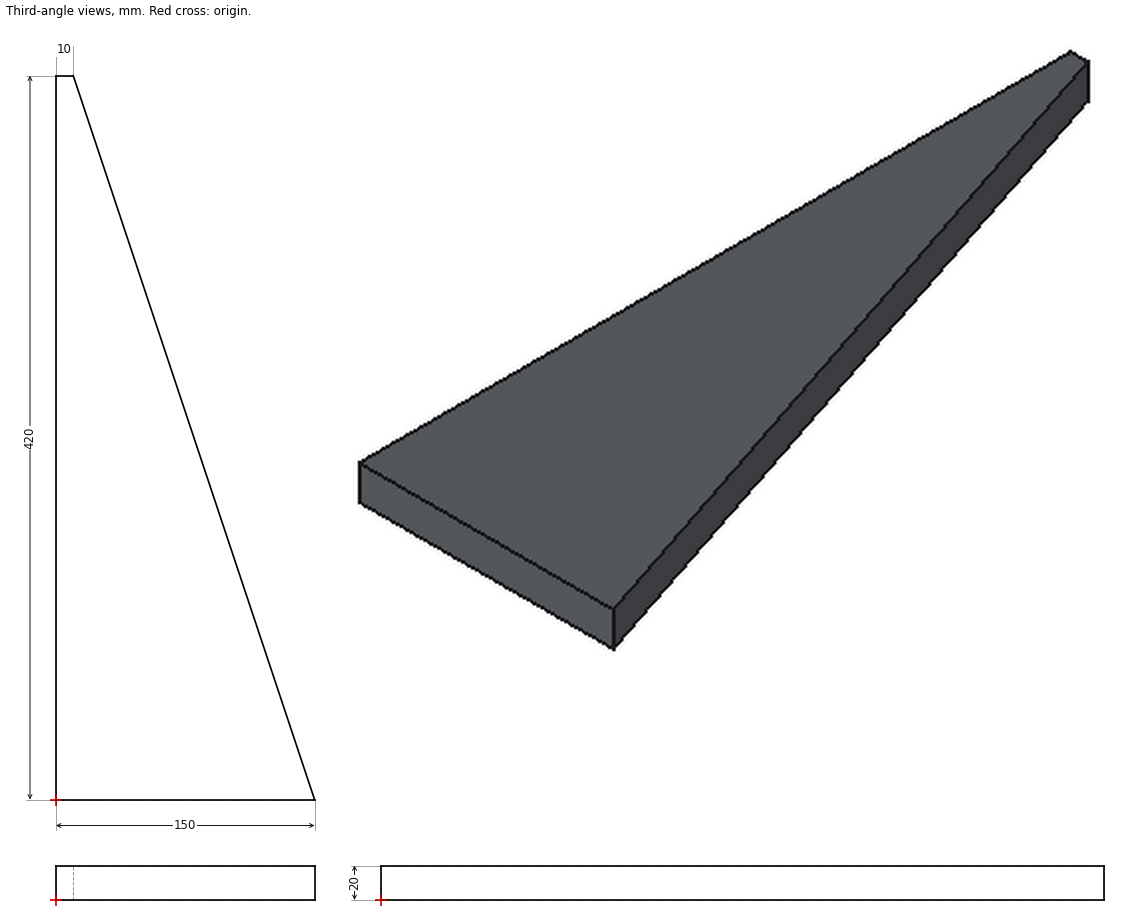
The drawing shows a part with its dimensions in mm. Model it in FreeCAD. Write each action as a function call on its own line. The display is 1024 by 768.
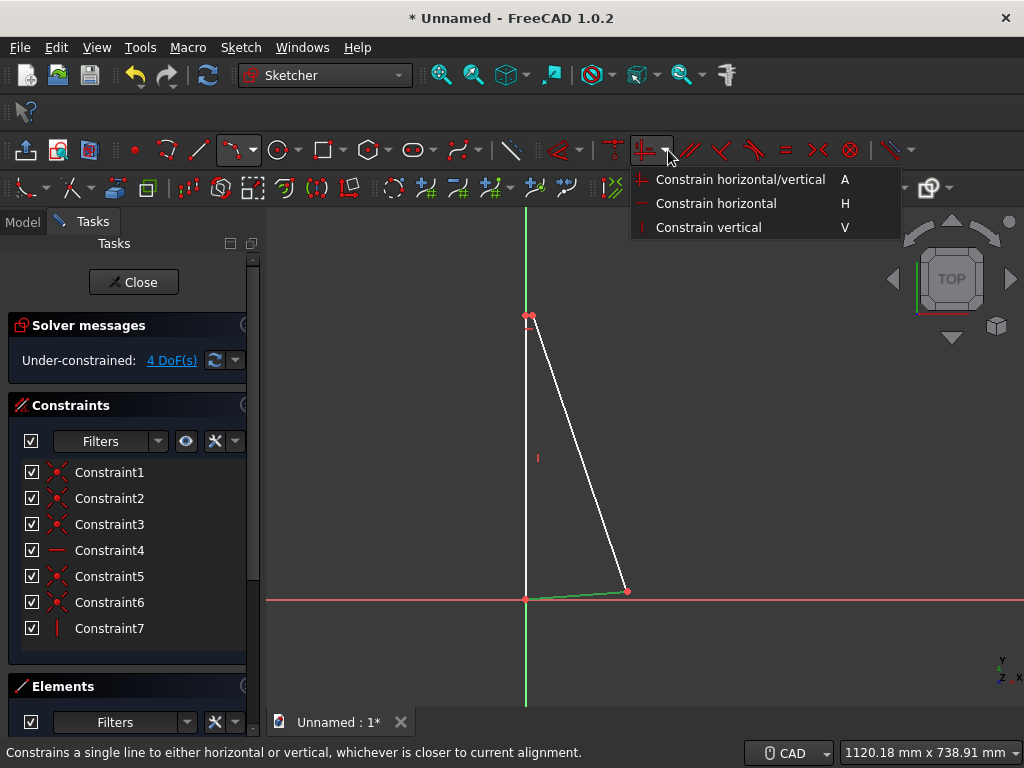
click(766, 203)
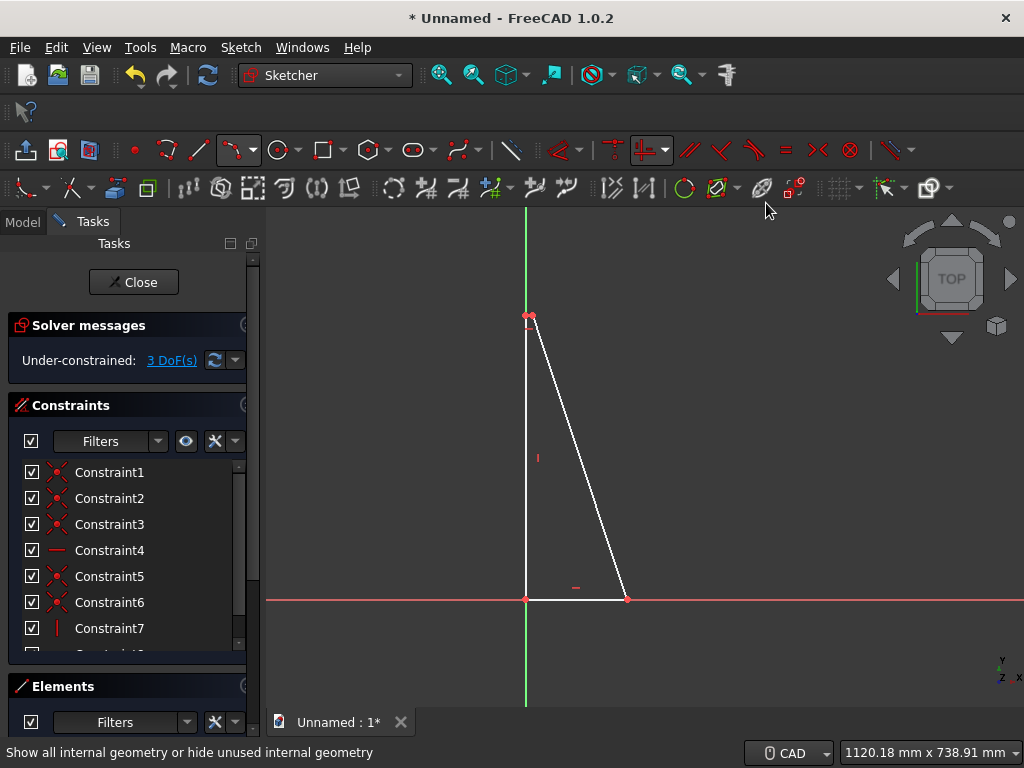
click(558, 150)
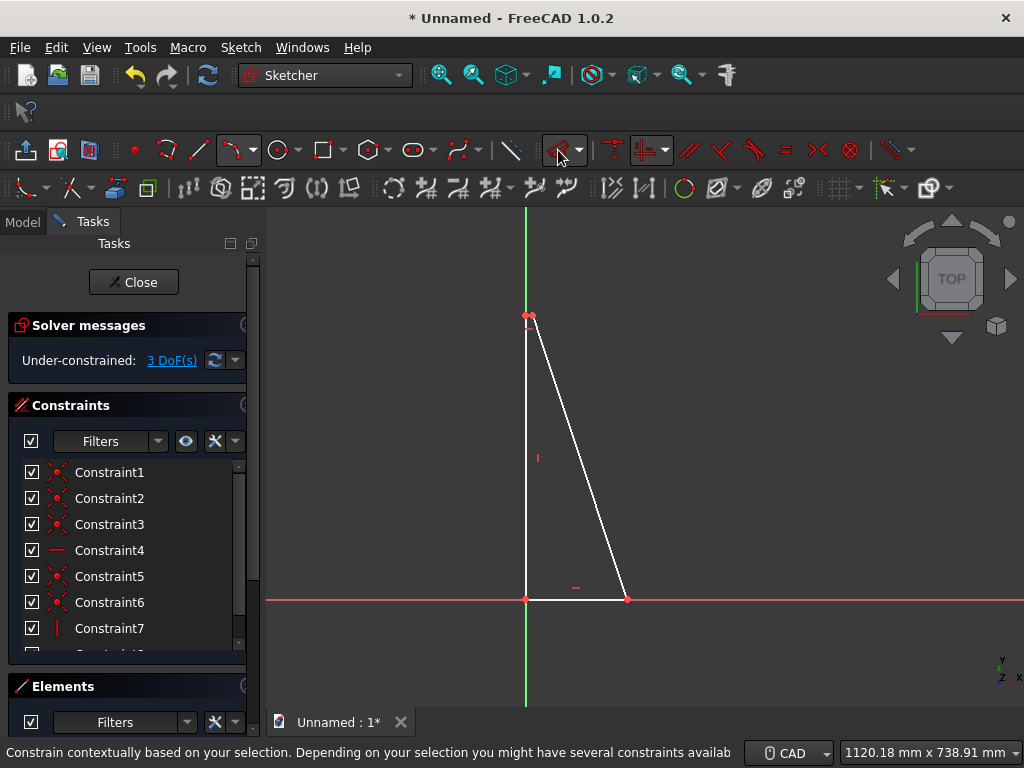
scroll(529, 316, up, 9)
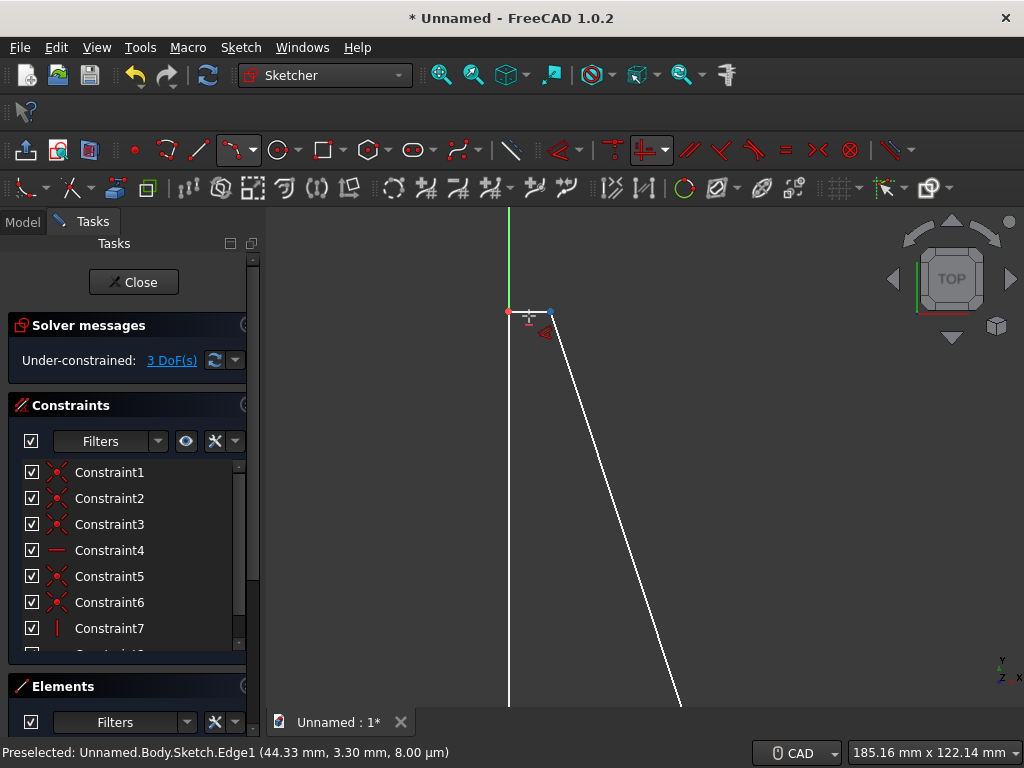
click(530, 312)
click(530, 278)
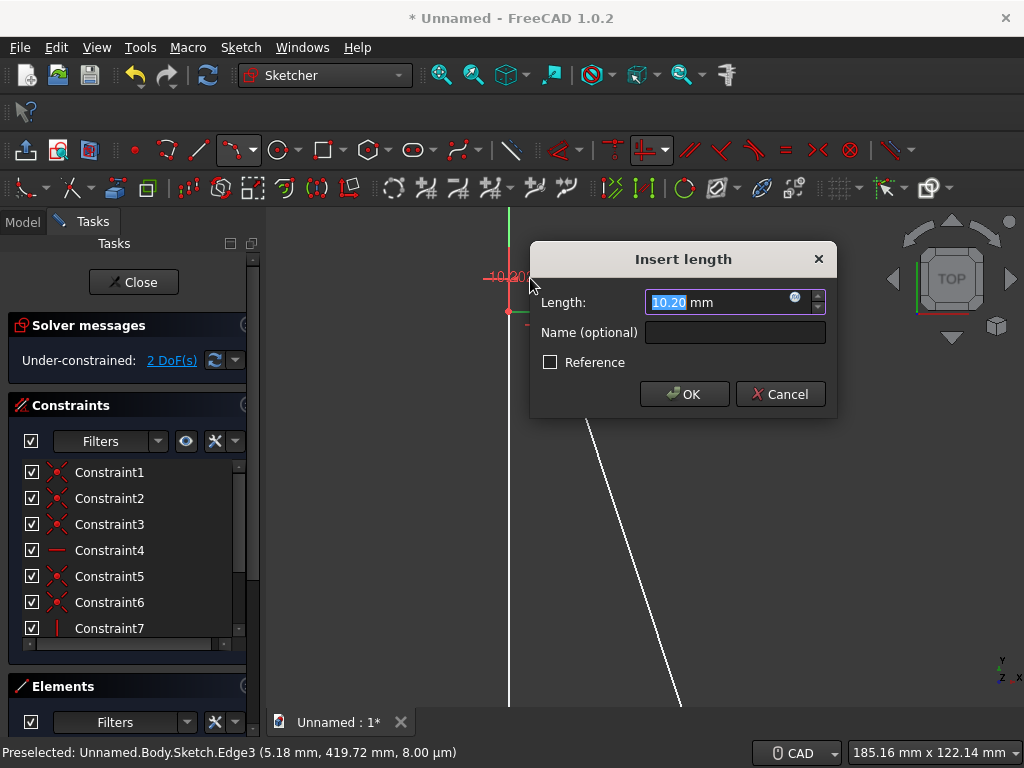
text(10)
key(Return)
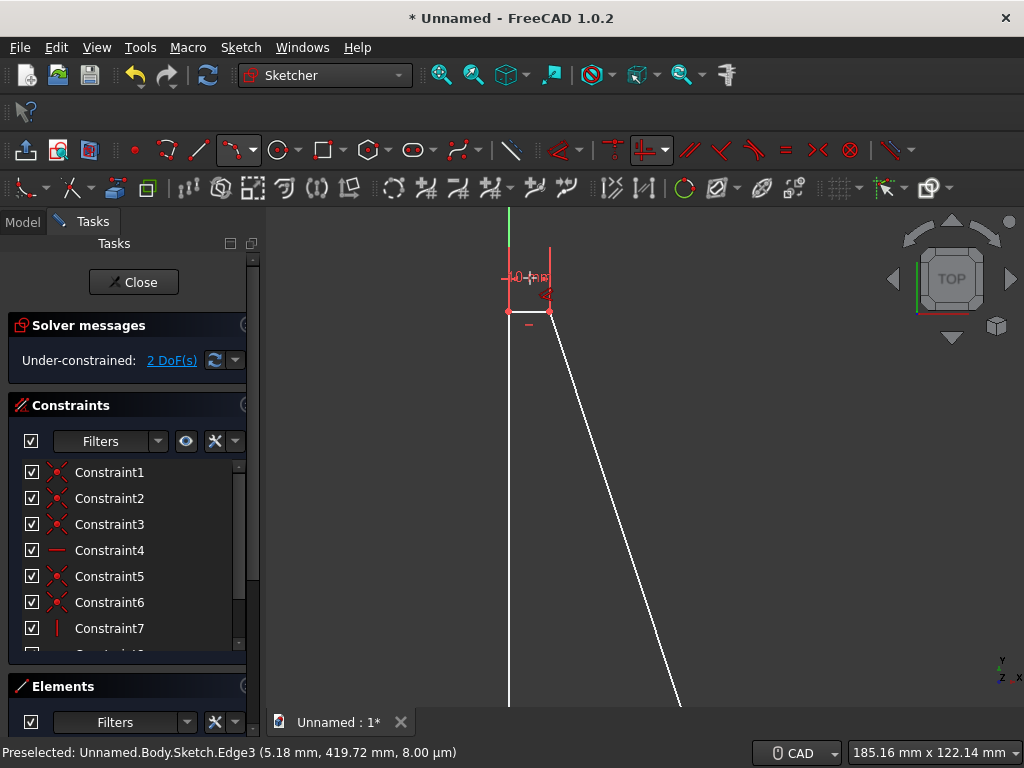
scroll(529, 316, down, 9)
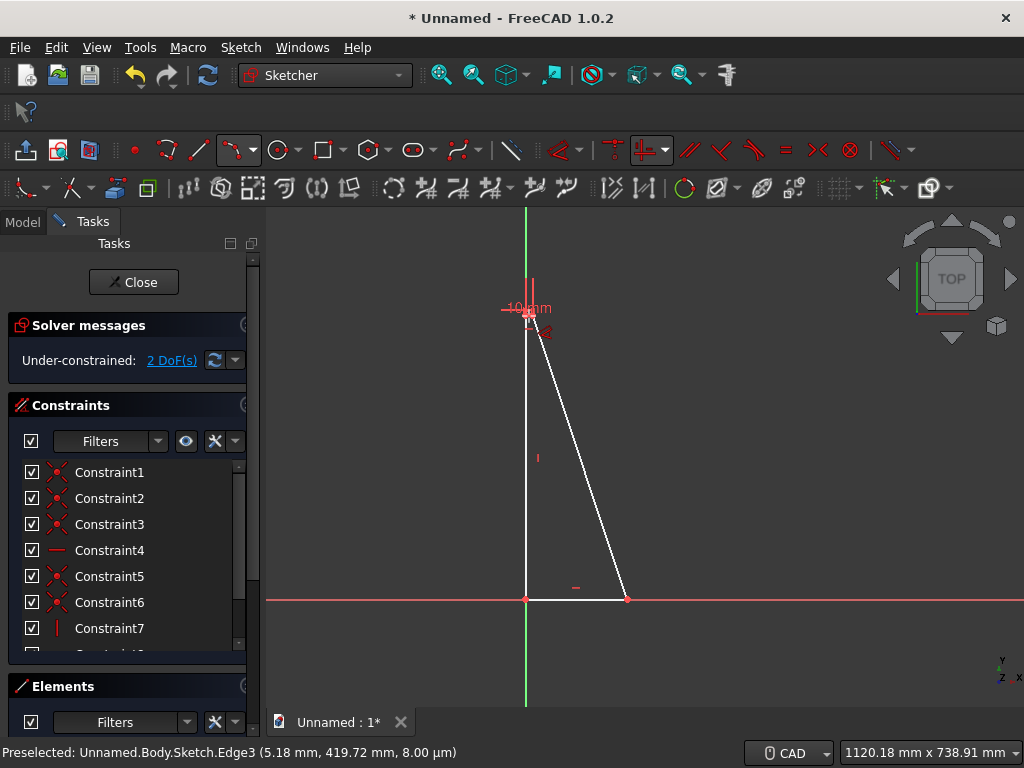
click(556, 600)
click(576, 634)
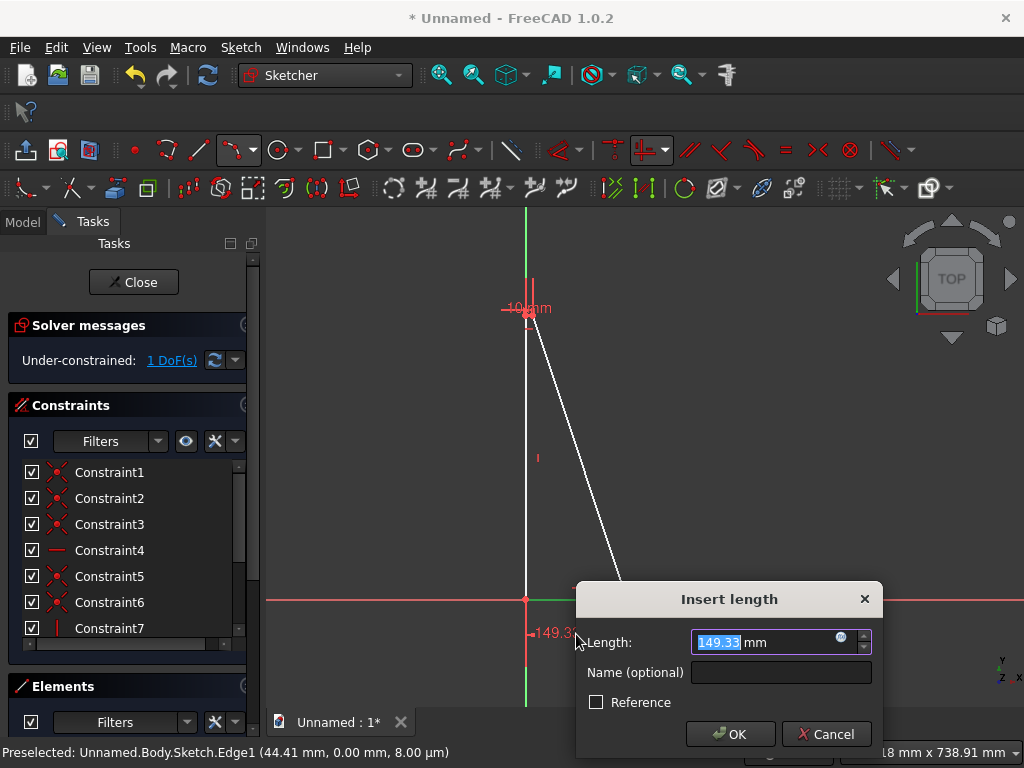
text(150)
key(Return)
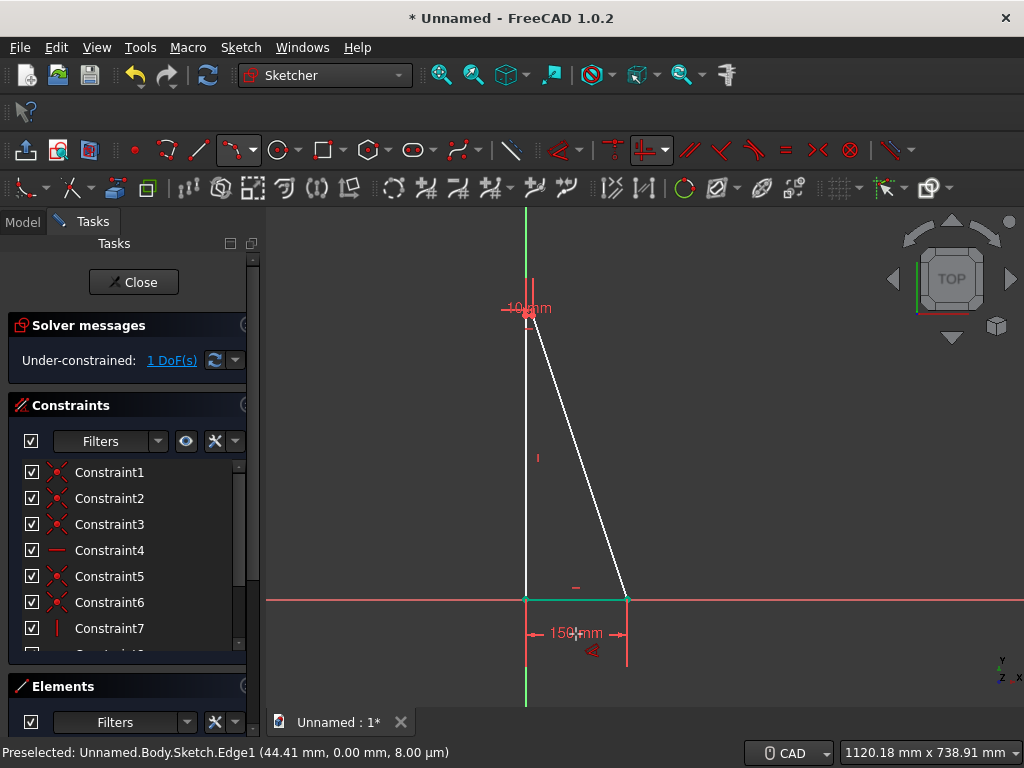
click(526, 401)
click(492, 458)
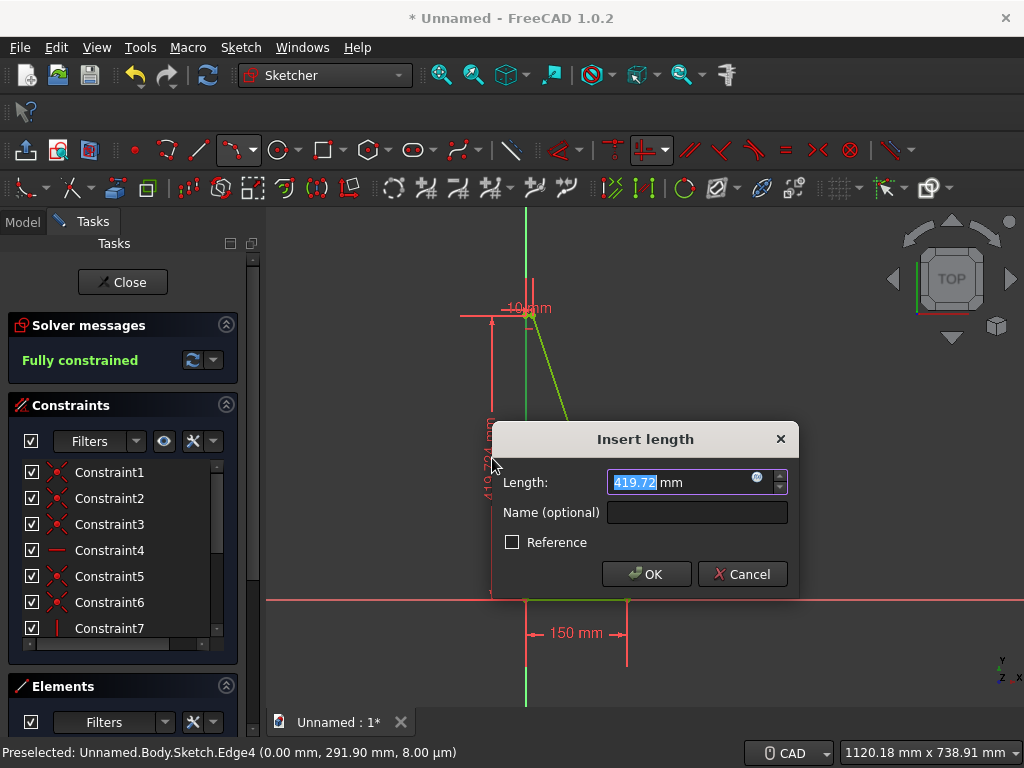
text(420)
key(Return)
key(Escape)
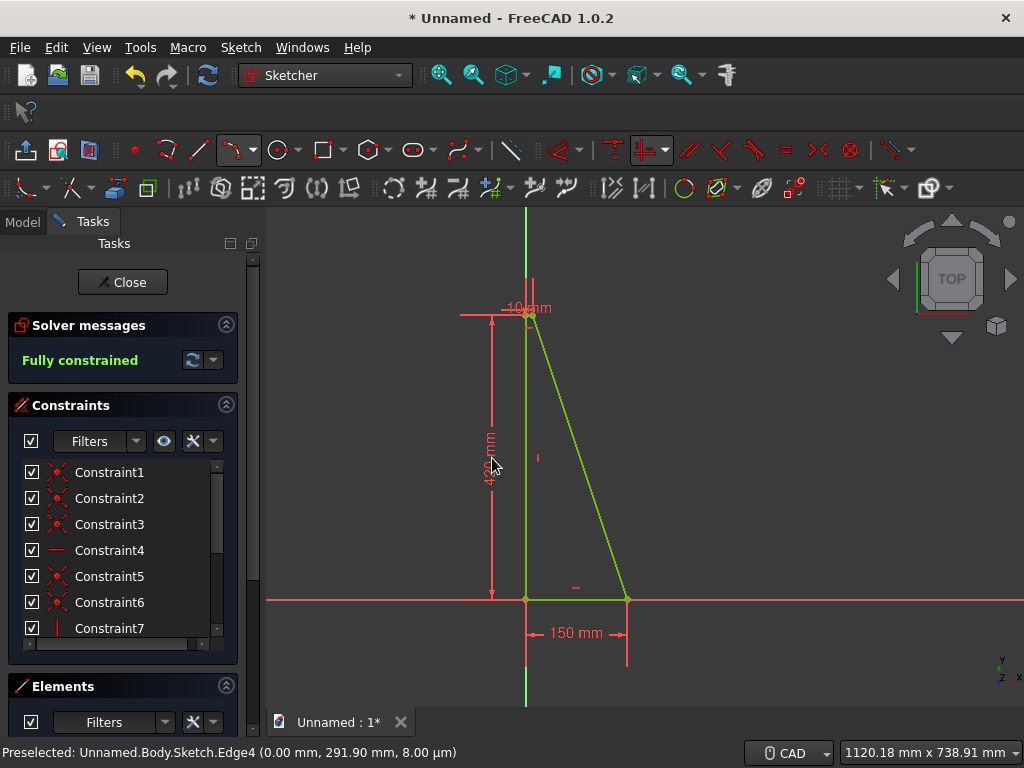
click(123, 282)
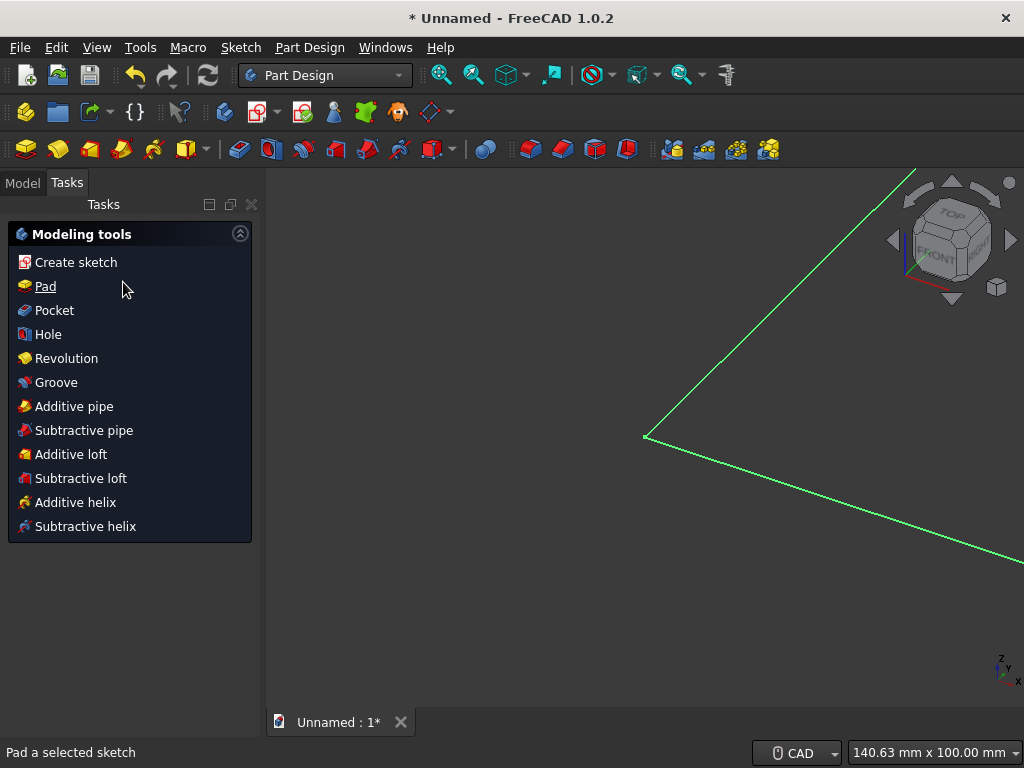
click(26, 150)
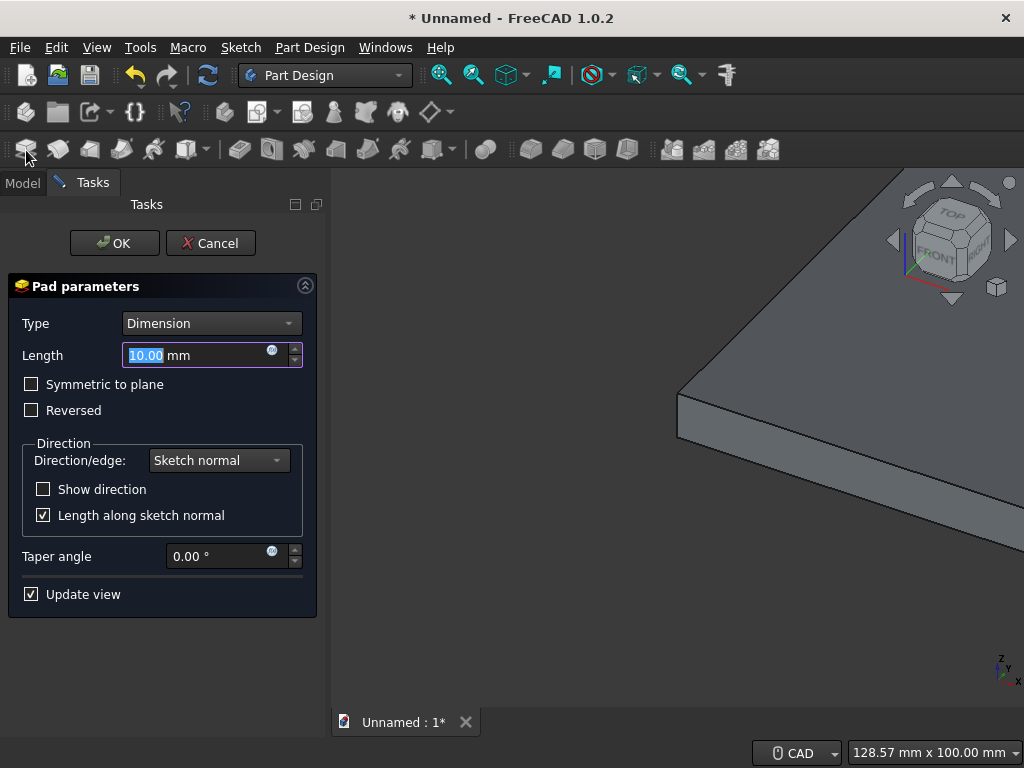
text(20)
key(Tab)